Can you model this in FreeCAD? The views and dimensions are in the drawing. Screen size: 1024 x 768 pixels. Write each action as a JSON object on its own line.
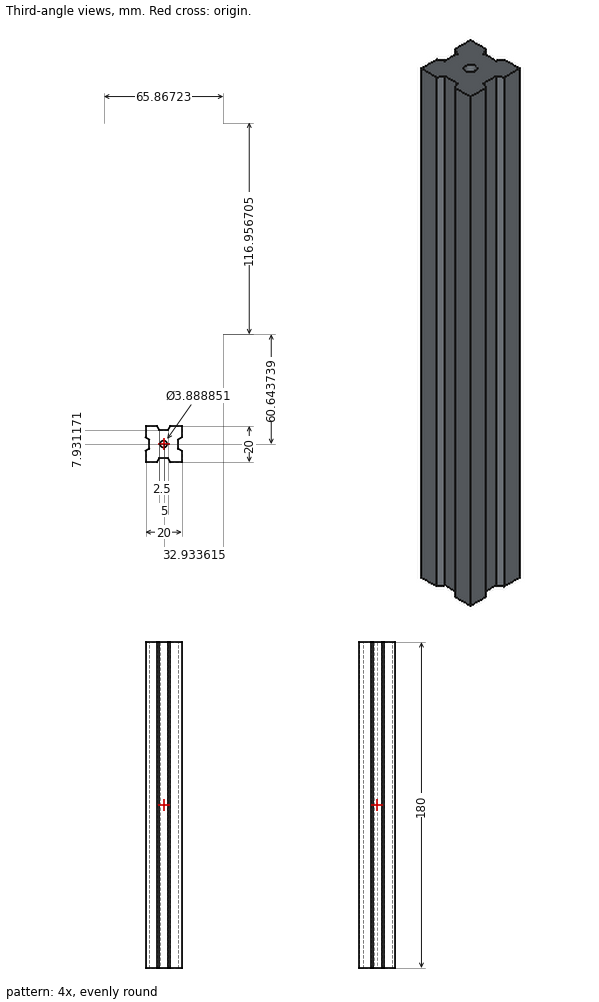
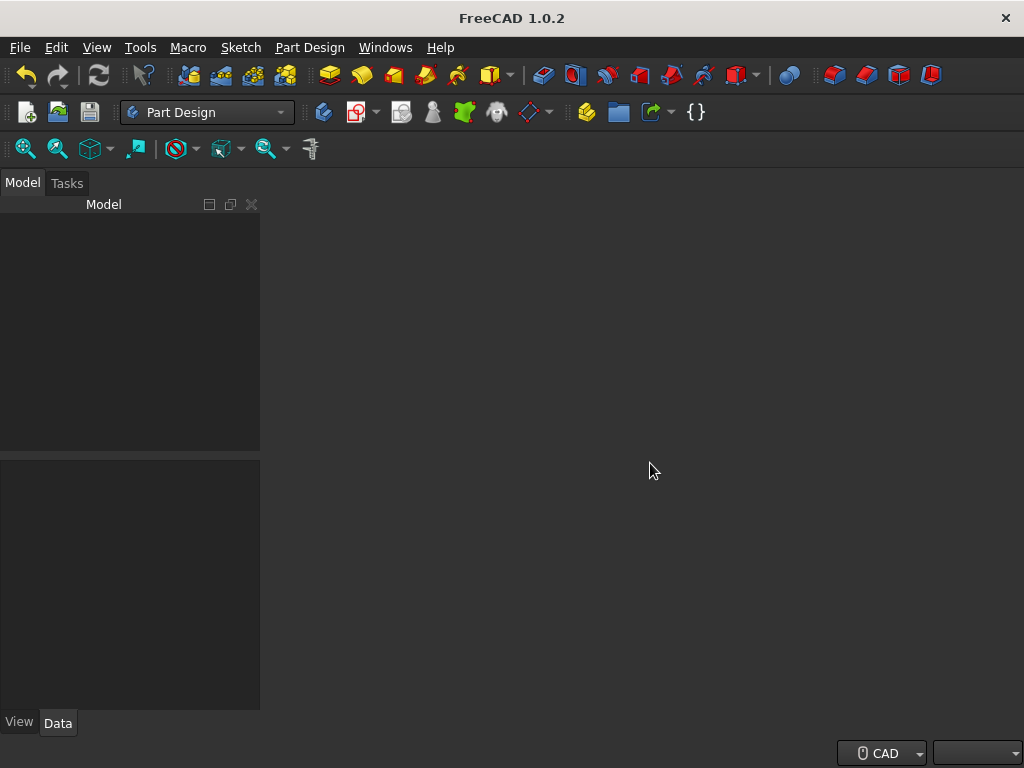
{"action": "left_click", "coordinate": [26, 112]}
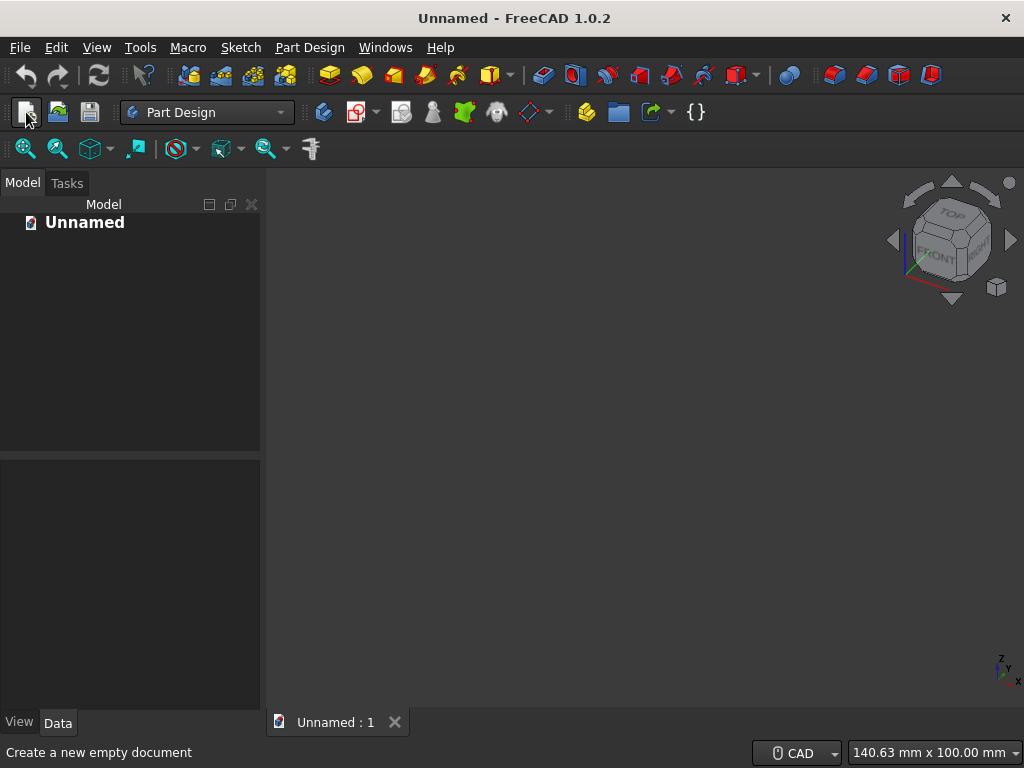
{"action": "left_click", "coordinate": [356, 112]}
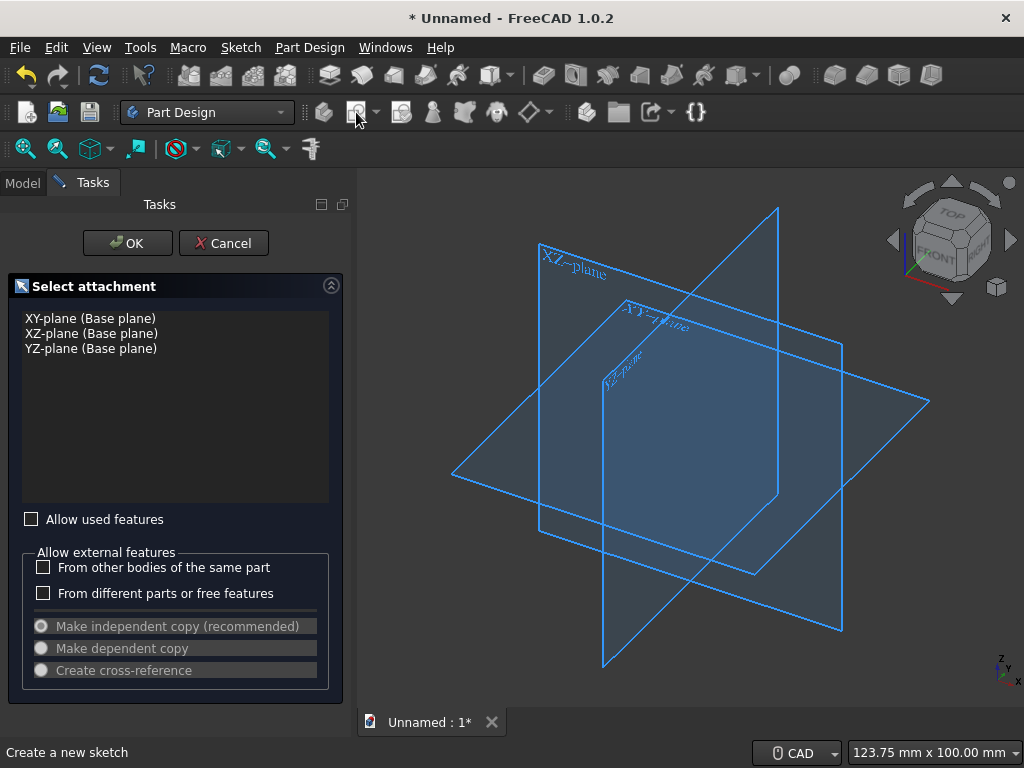
{"action": "left_click", "coordinate": [82, 318]}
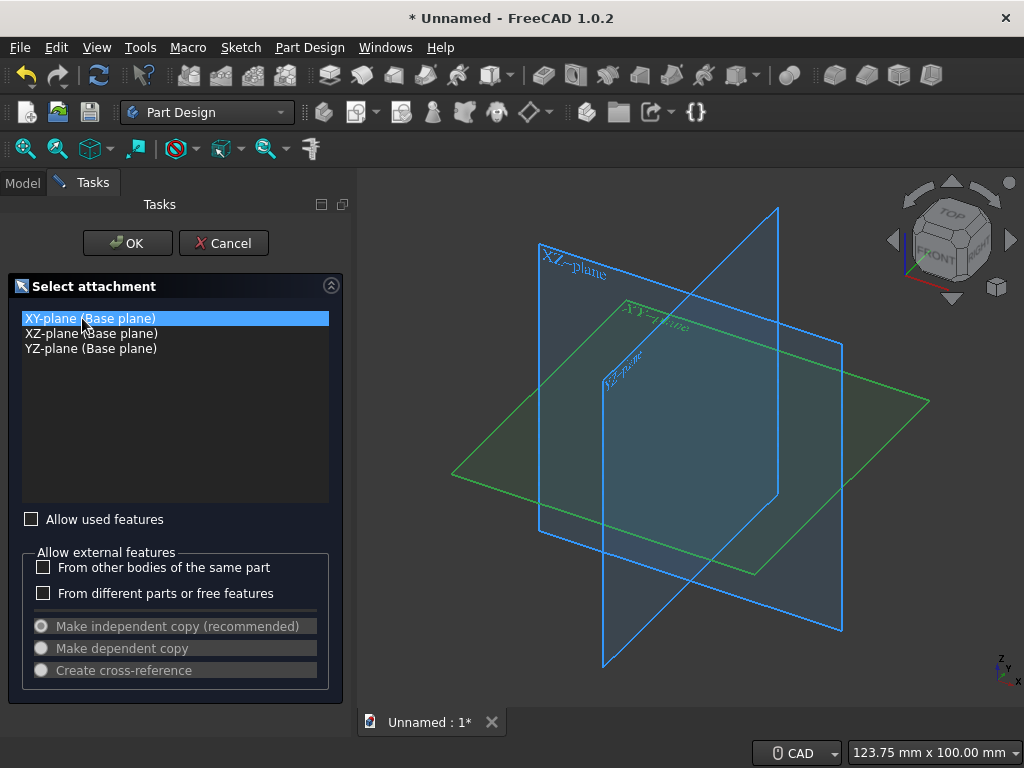
{"action": "left_click", "coordinate": [128, 243]}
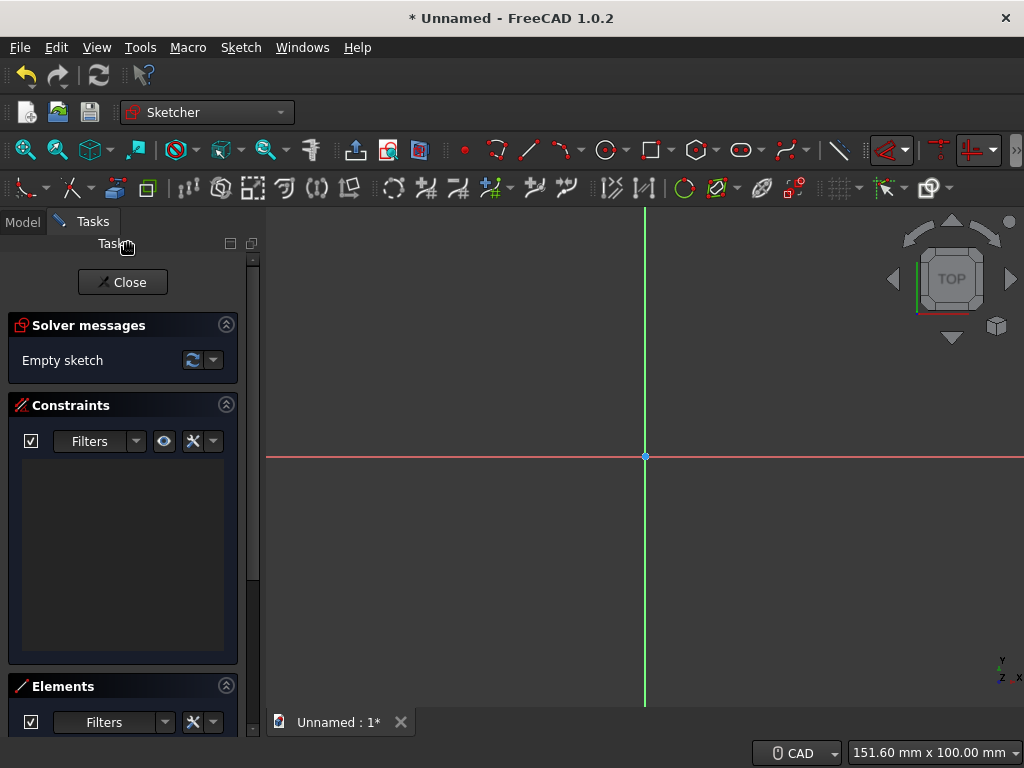
{"action": "scroll", "coordinate": [675, 457], "scroll_direction": "up", "scroll_amount": 6}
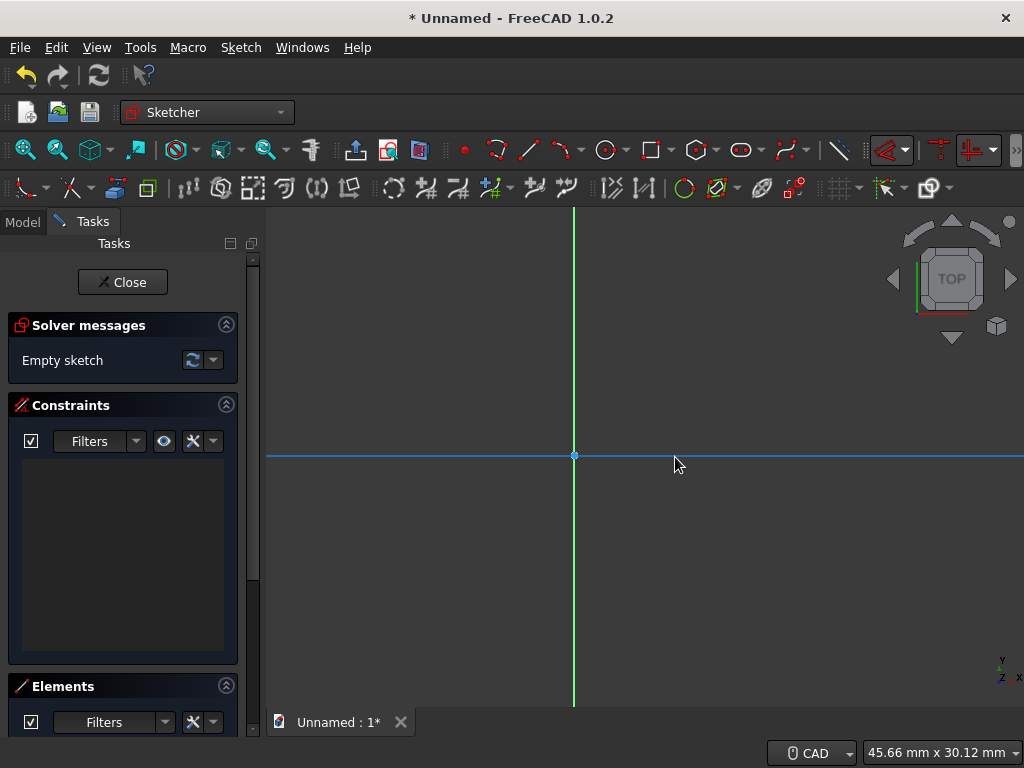
{"action": "key", "text": "g v"}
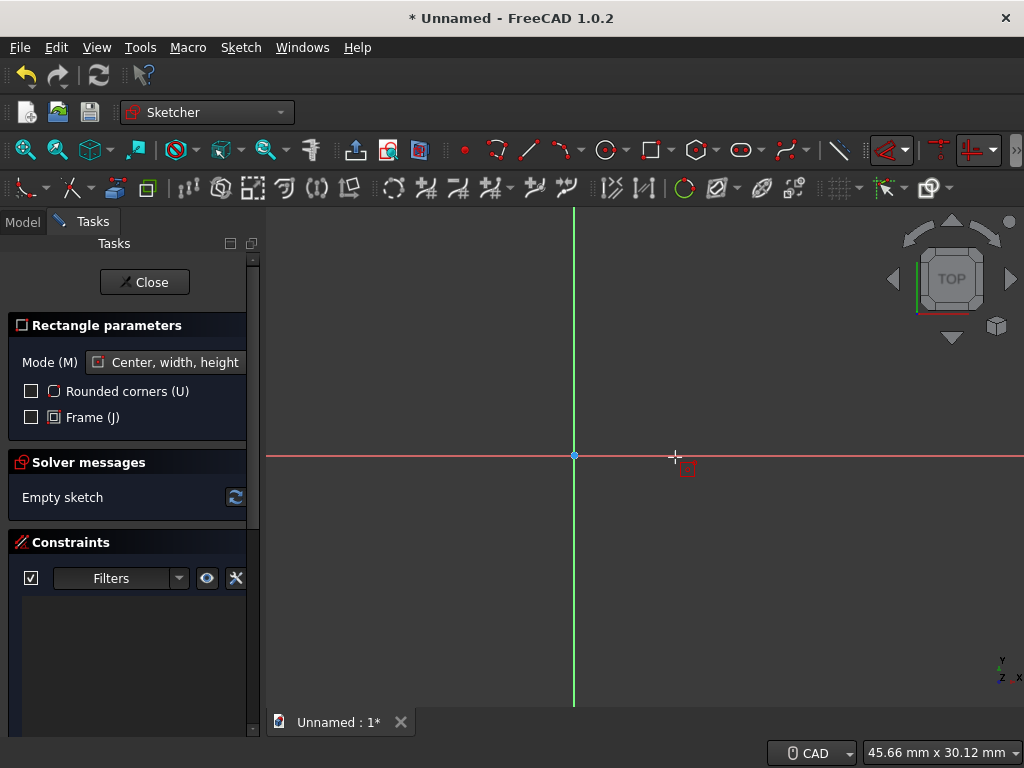
{"action": "left_click", "coordinate": [574, 456]}
{"action": "mouse_move", "coordinate": [740, 290]}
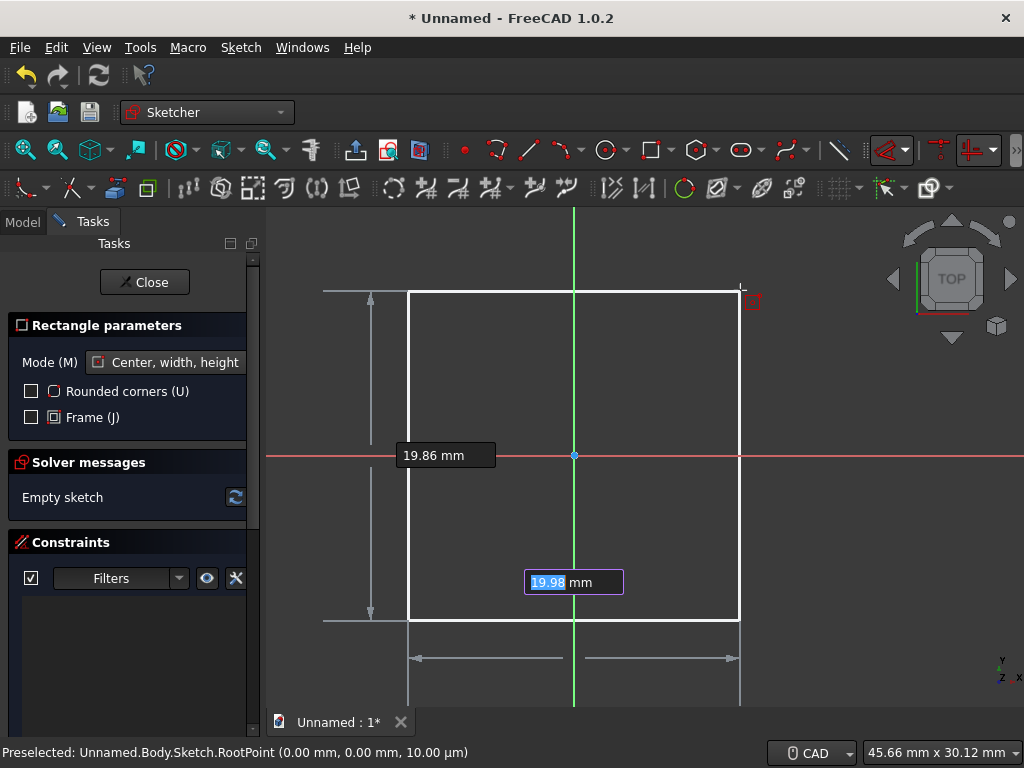
{"action": "type", "text": "20"}
{"action": "key", "text": "Tab"}
{"action": "type", "text": "20"}
{"action": "key", "text": "Return"}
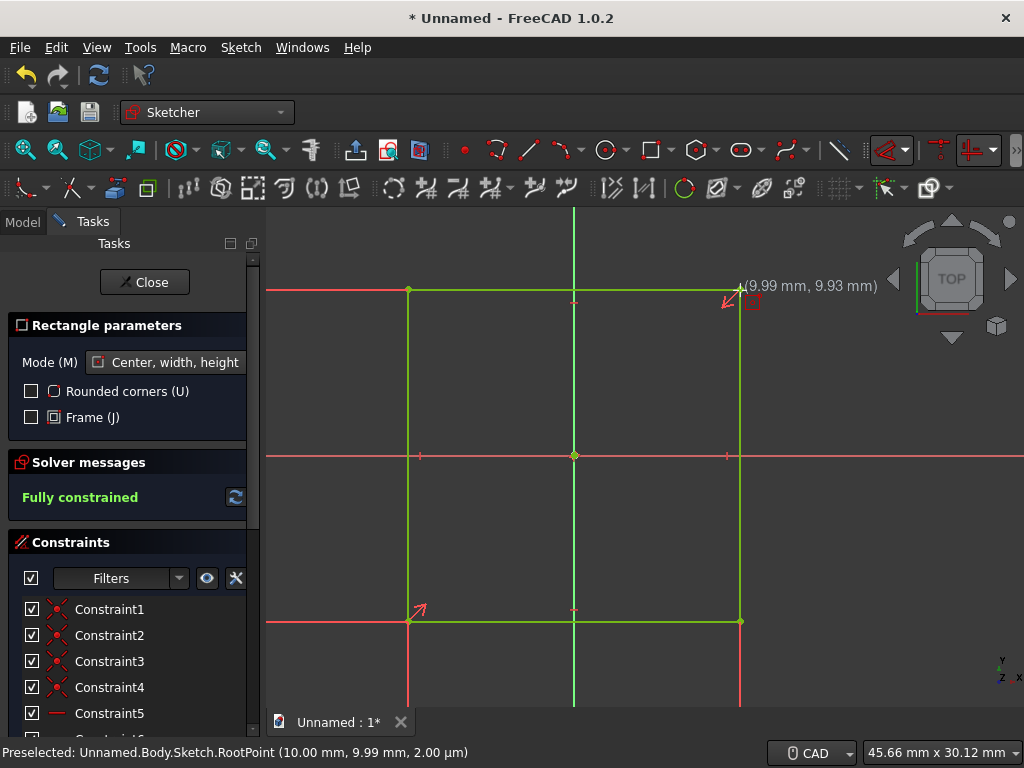
{"action": "left_click", "coordinate": [606, 150]}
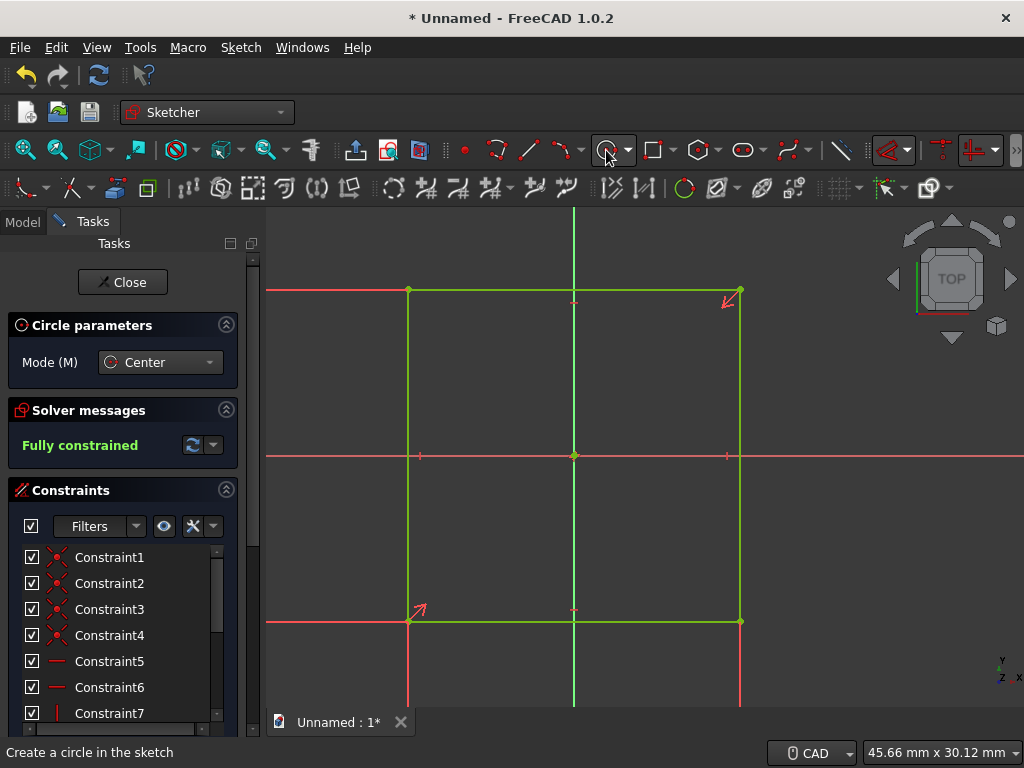
{"action": "left_click", "coordinate": [574, 456]}
{"action": "mouse_move", "coordinate": [597, 433]}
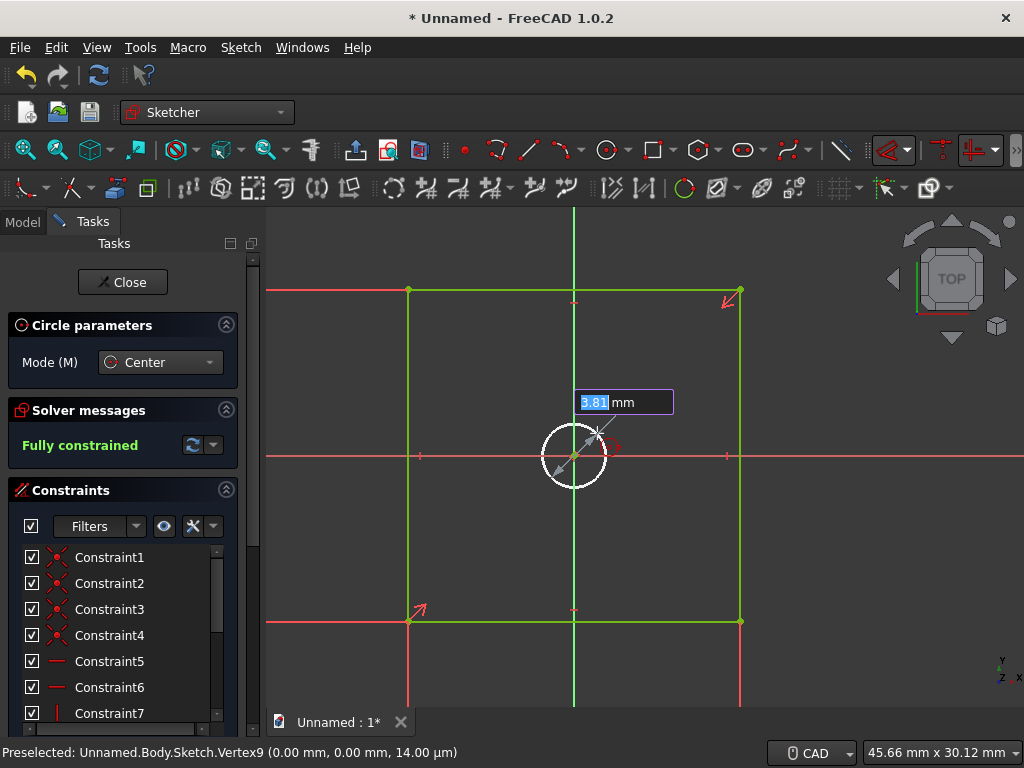
{"action": "type", "text": "3.888851"}
{"action": "key", "text": "Return"}
{"action": "key", "text": "Escape"}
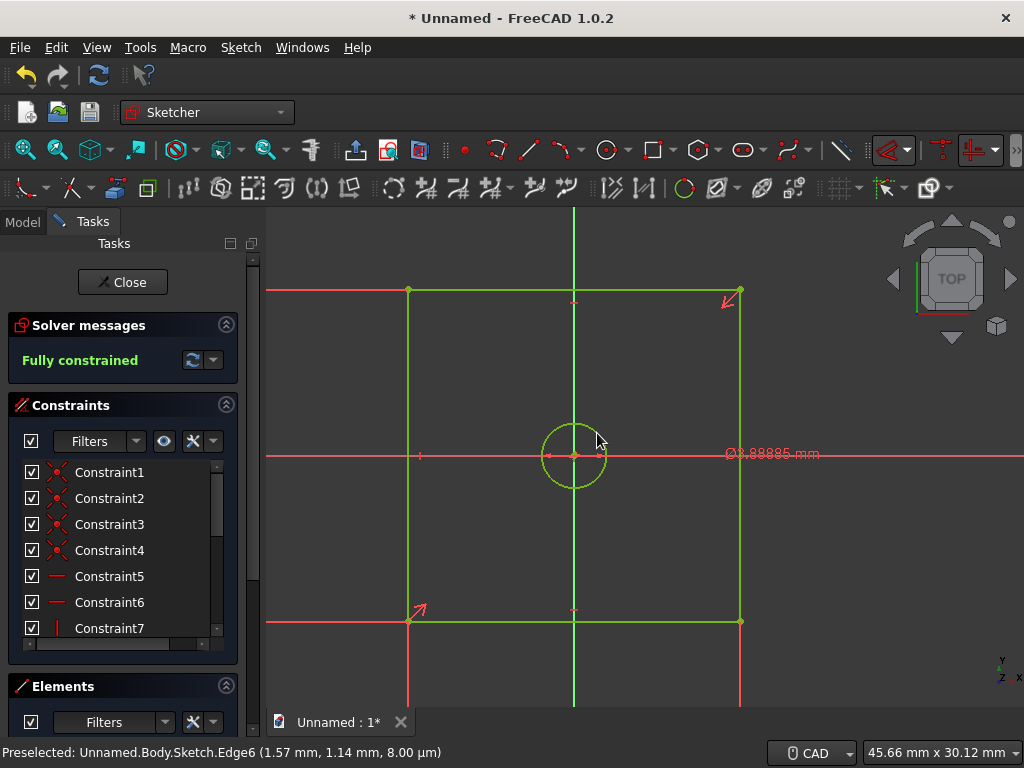
{"action": "left_click", "coordinate": [123, 282]}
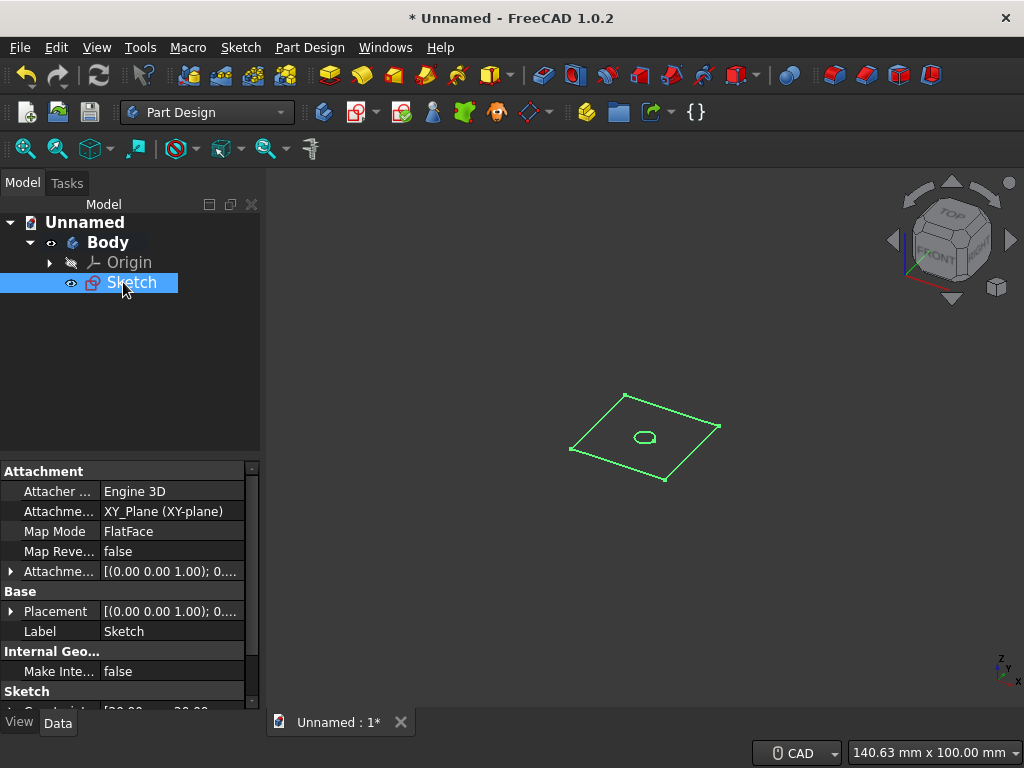
{"action": "left_click", "coordinate": [330, 76]}